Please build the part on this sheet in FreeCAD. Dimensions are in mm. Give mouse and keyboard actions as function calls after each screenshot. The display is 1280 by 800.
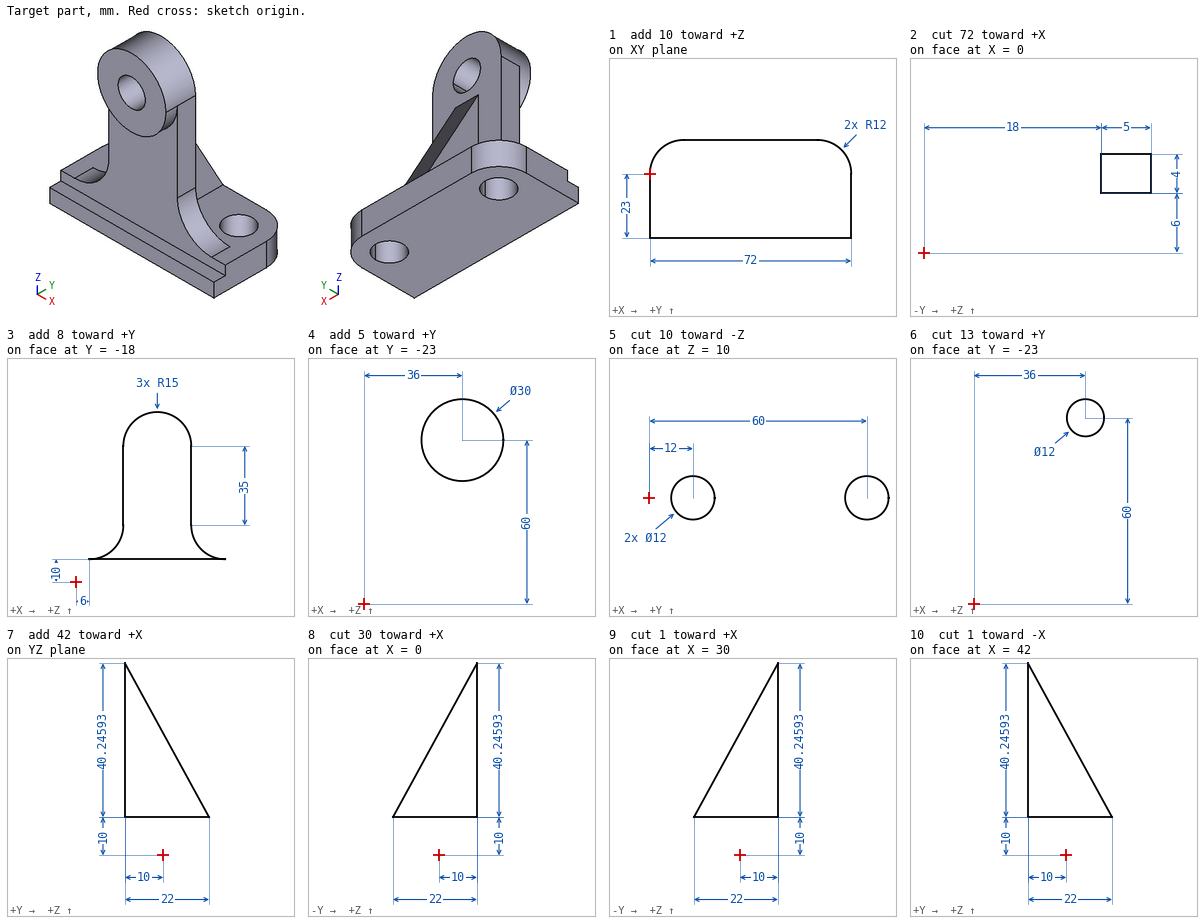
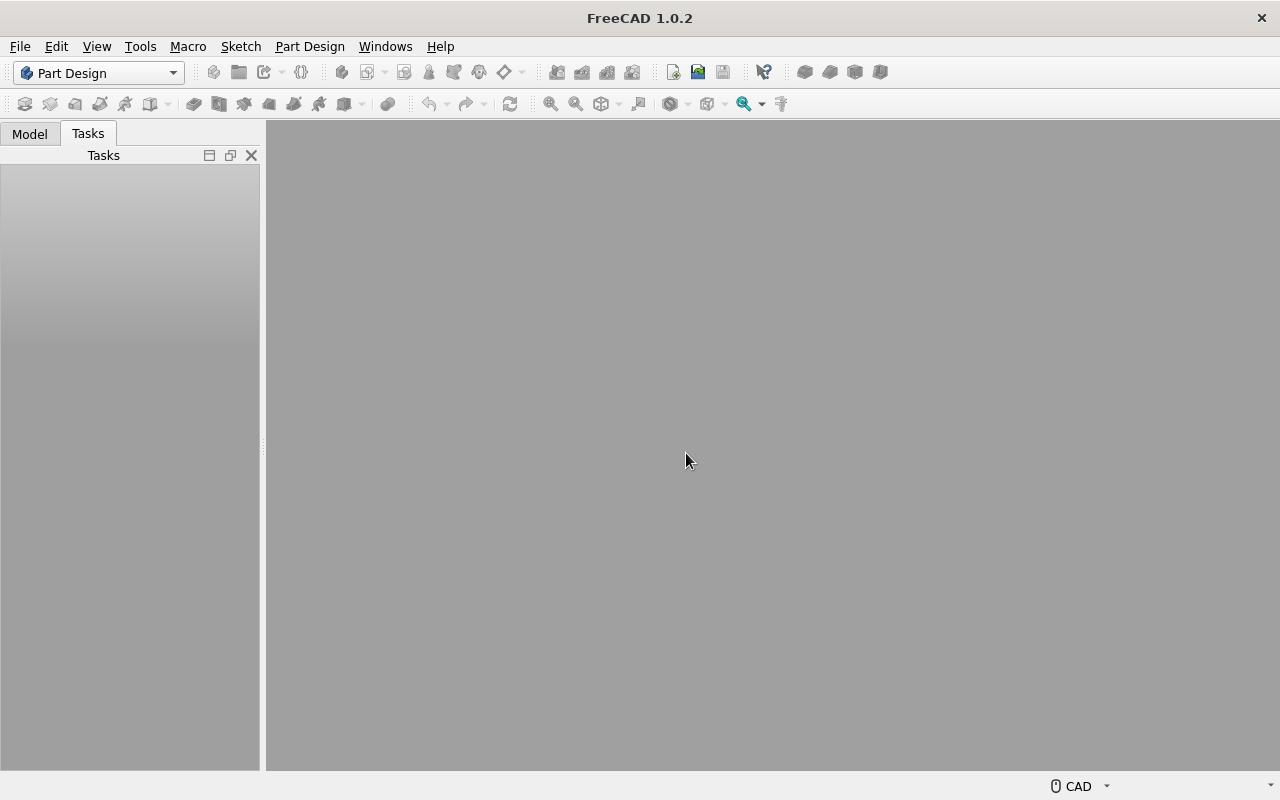
click(673, 72)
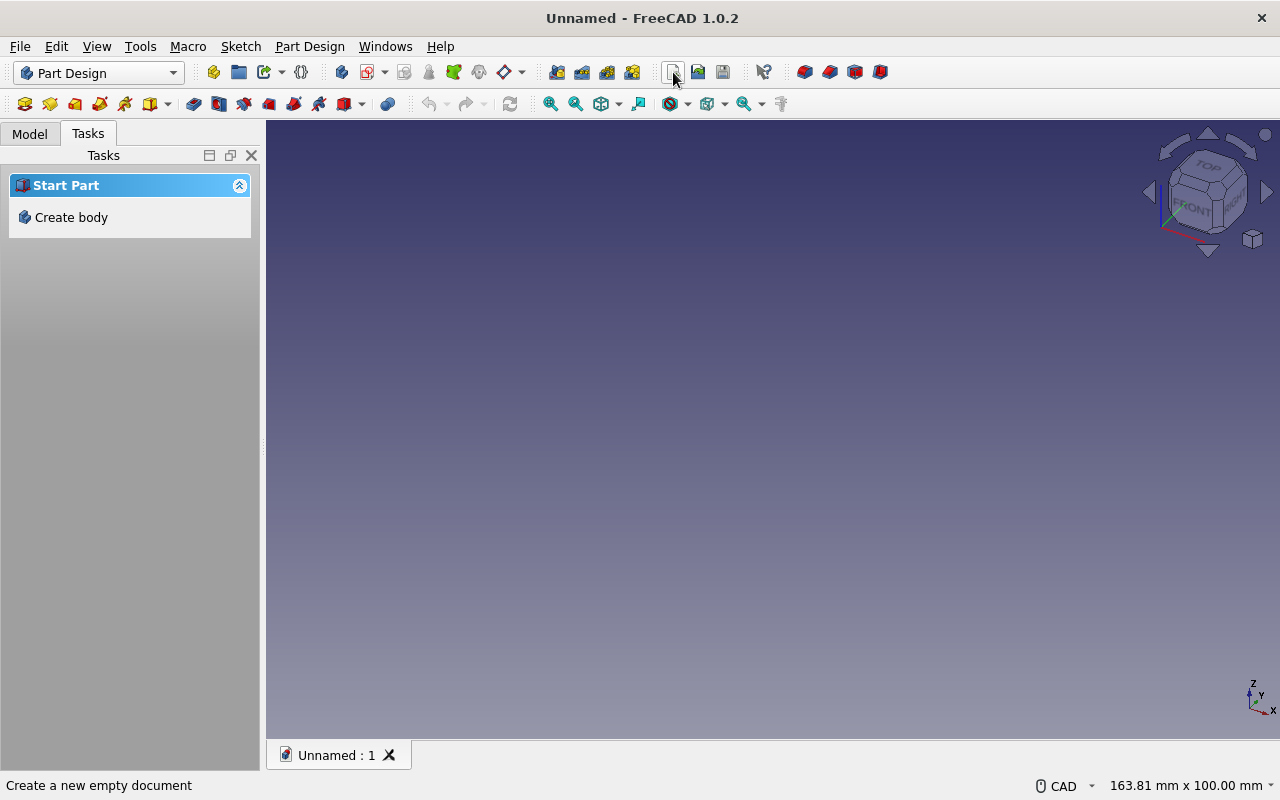
click(366, 72)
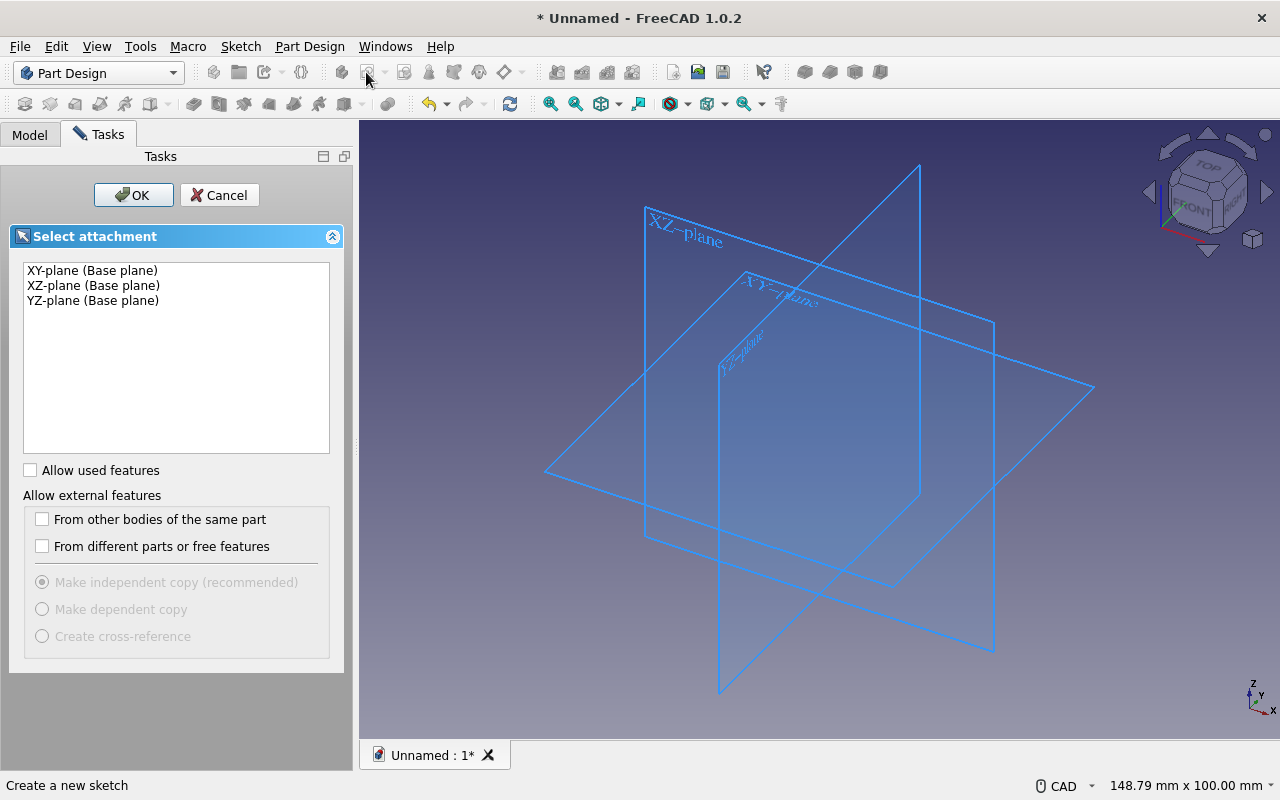
click(84, 270)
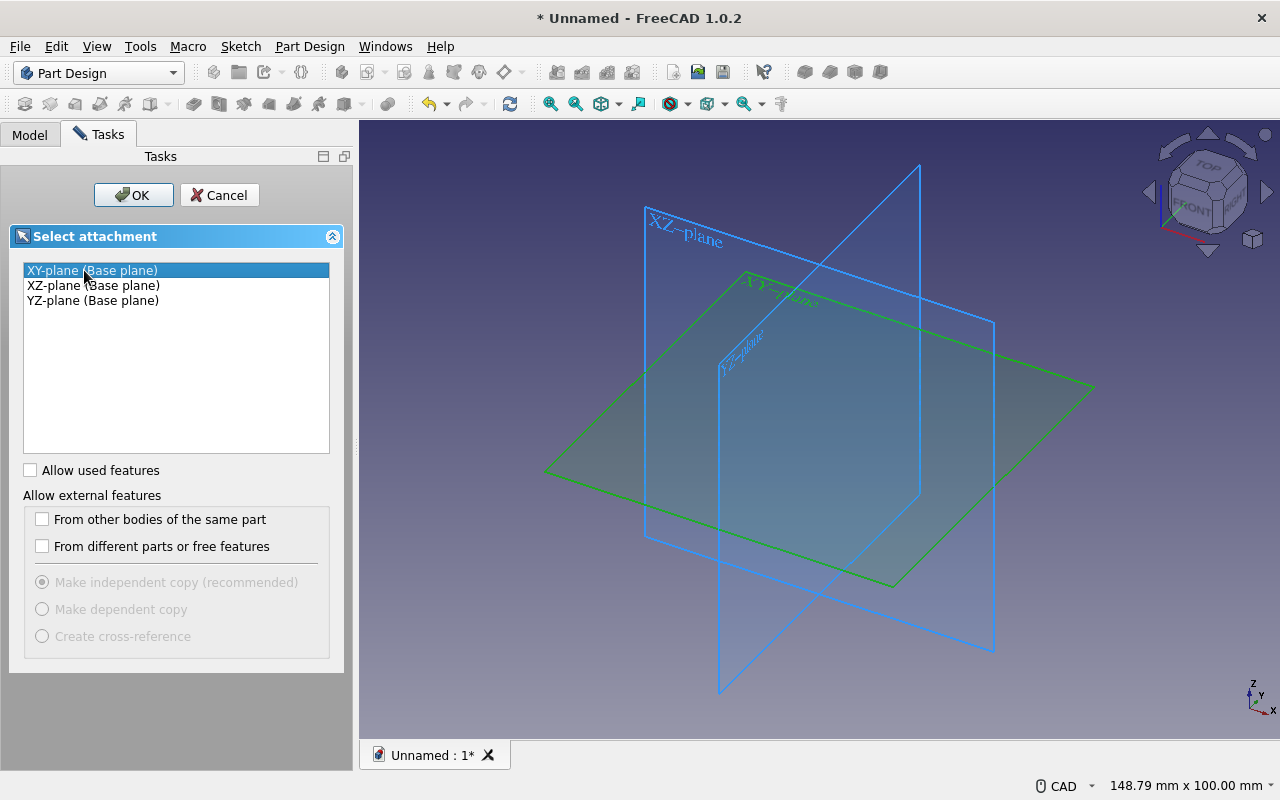
click(134, 195)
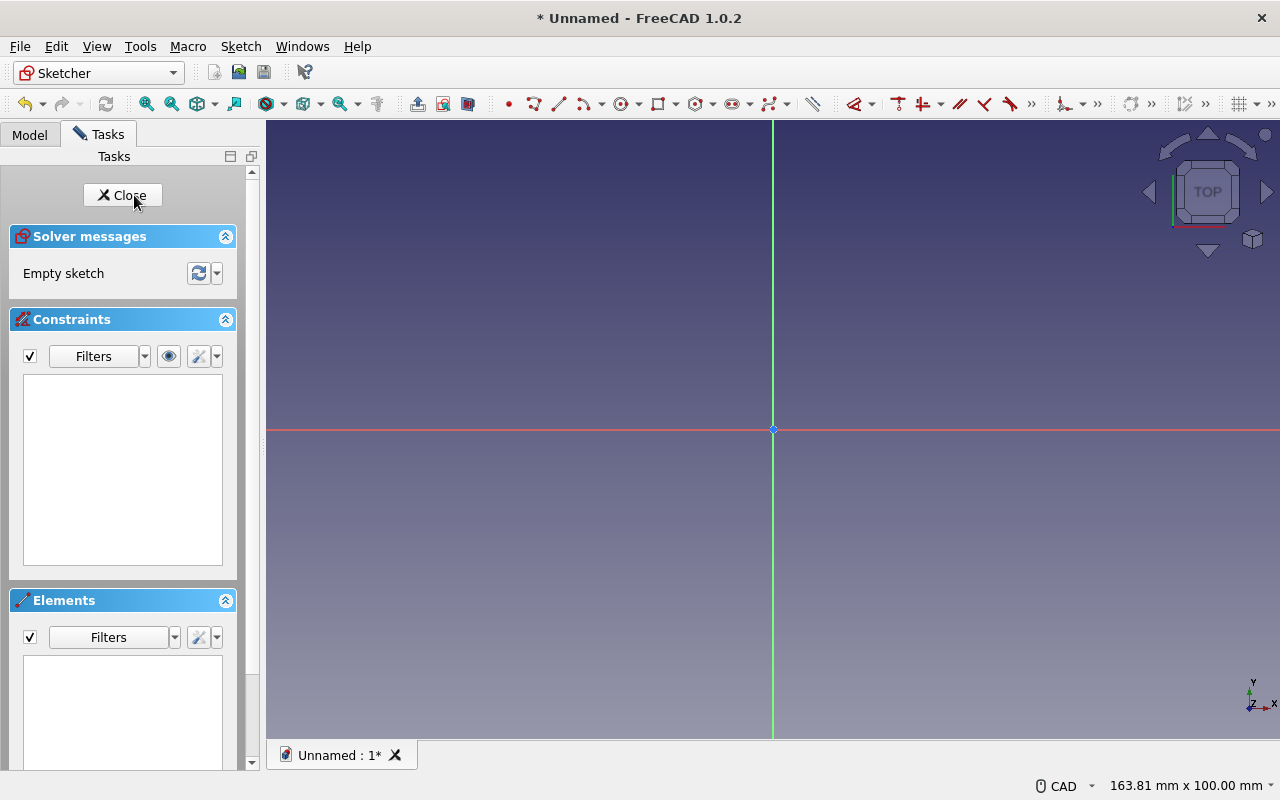
scroll(294, 276, down, 1)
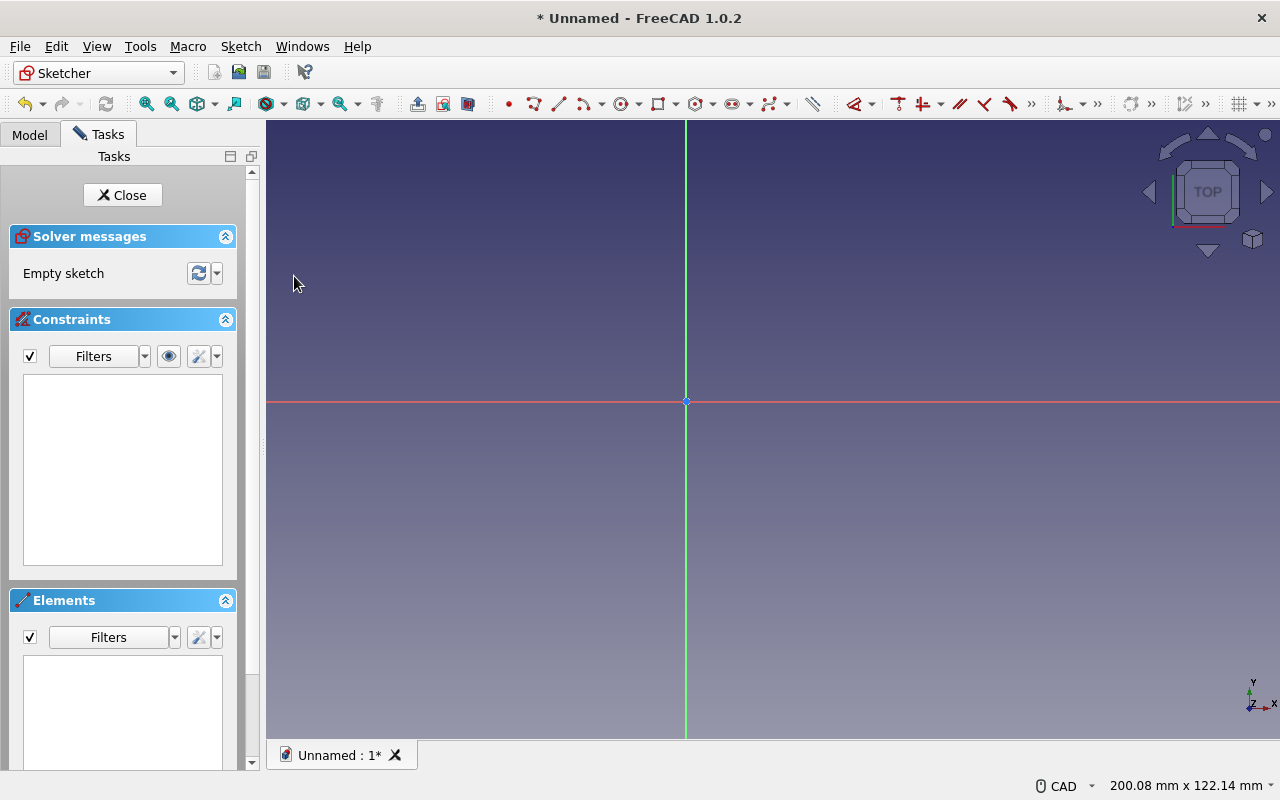
scroll(1115, 430, up, 2)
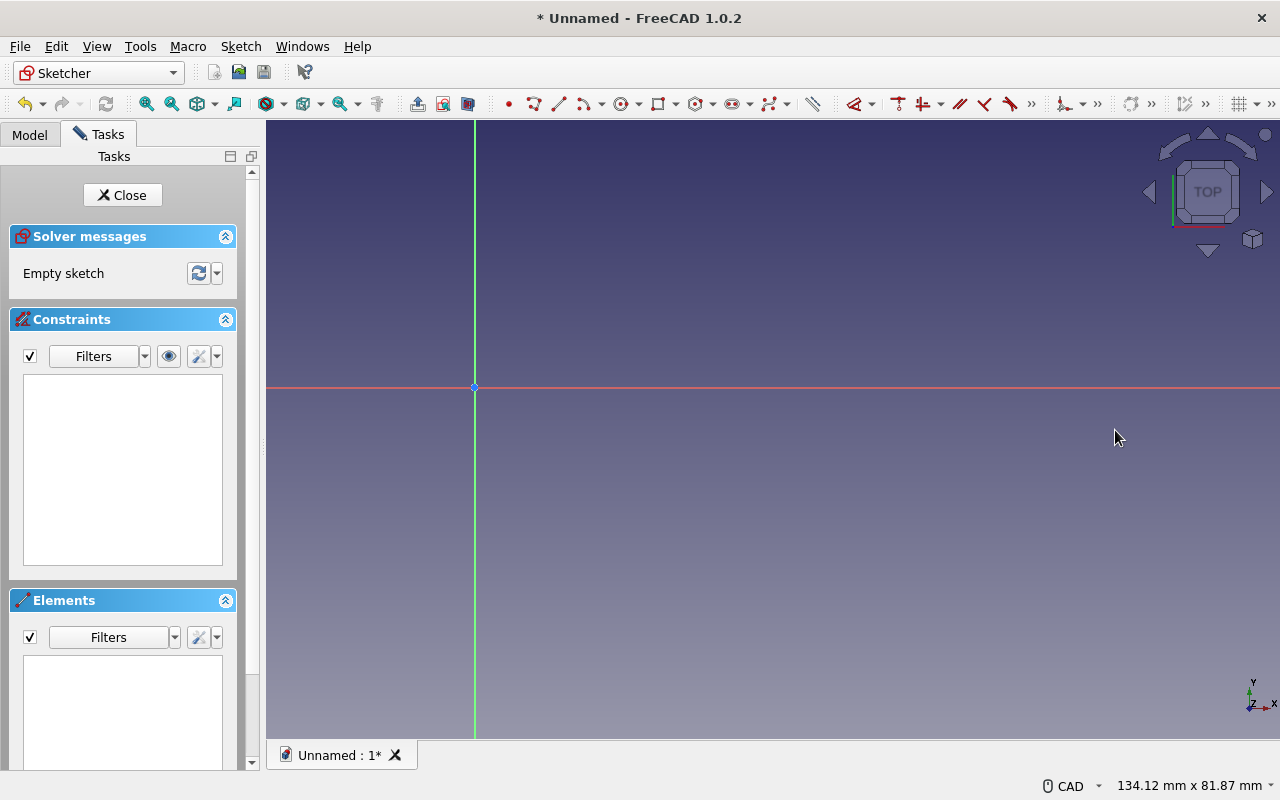
key(g)
key(m)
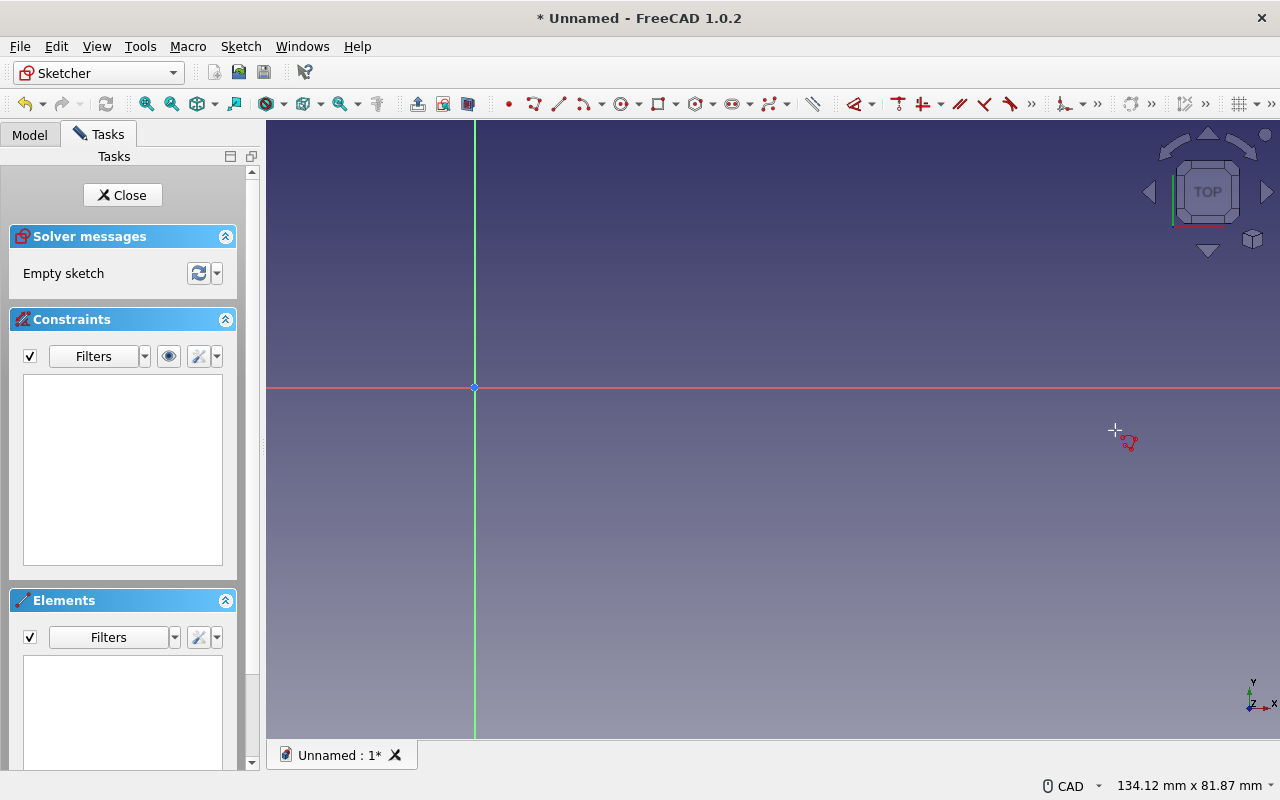
click(475, 388)
click(484, 561)
click(1019, 561)
click(1019, 388)
right_click(1019, 388)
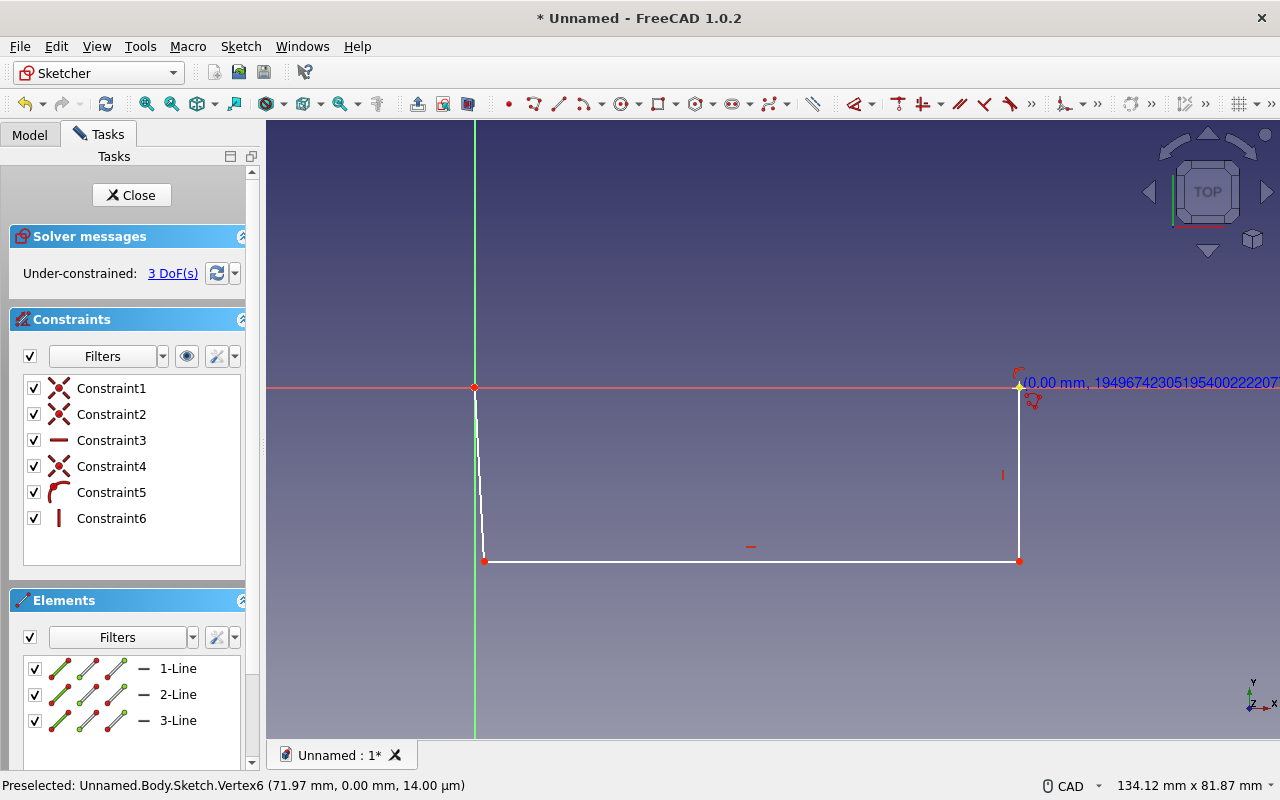
click(559, 104)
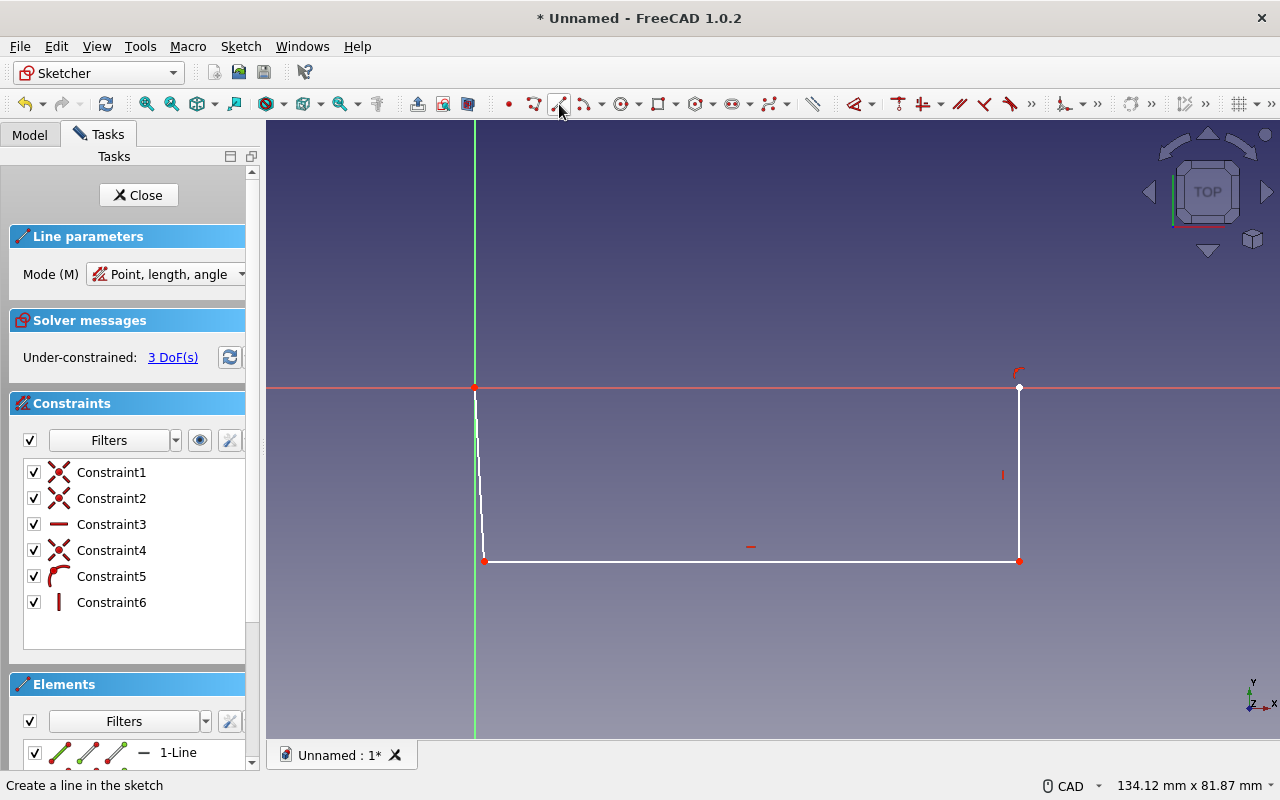
click(928, 297)
click(566, 297)